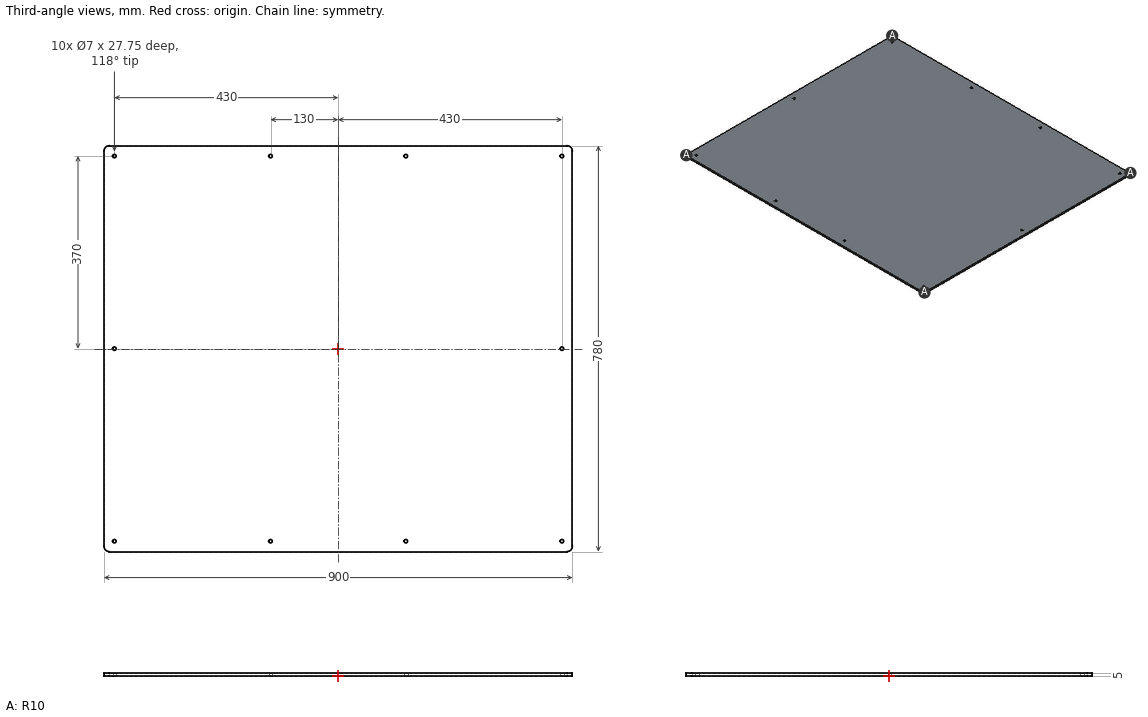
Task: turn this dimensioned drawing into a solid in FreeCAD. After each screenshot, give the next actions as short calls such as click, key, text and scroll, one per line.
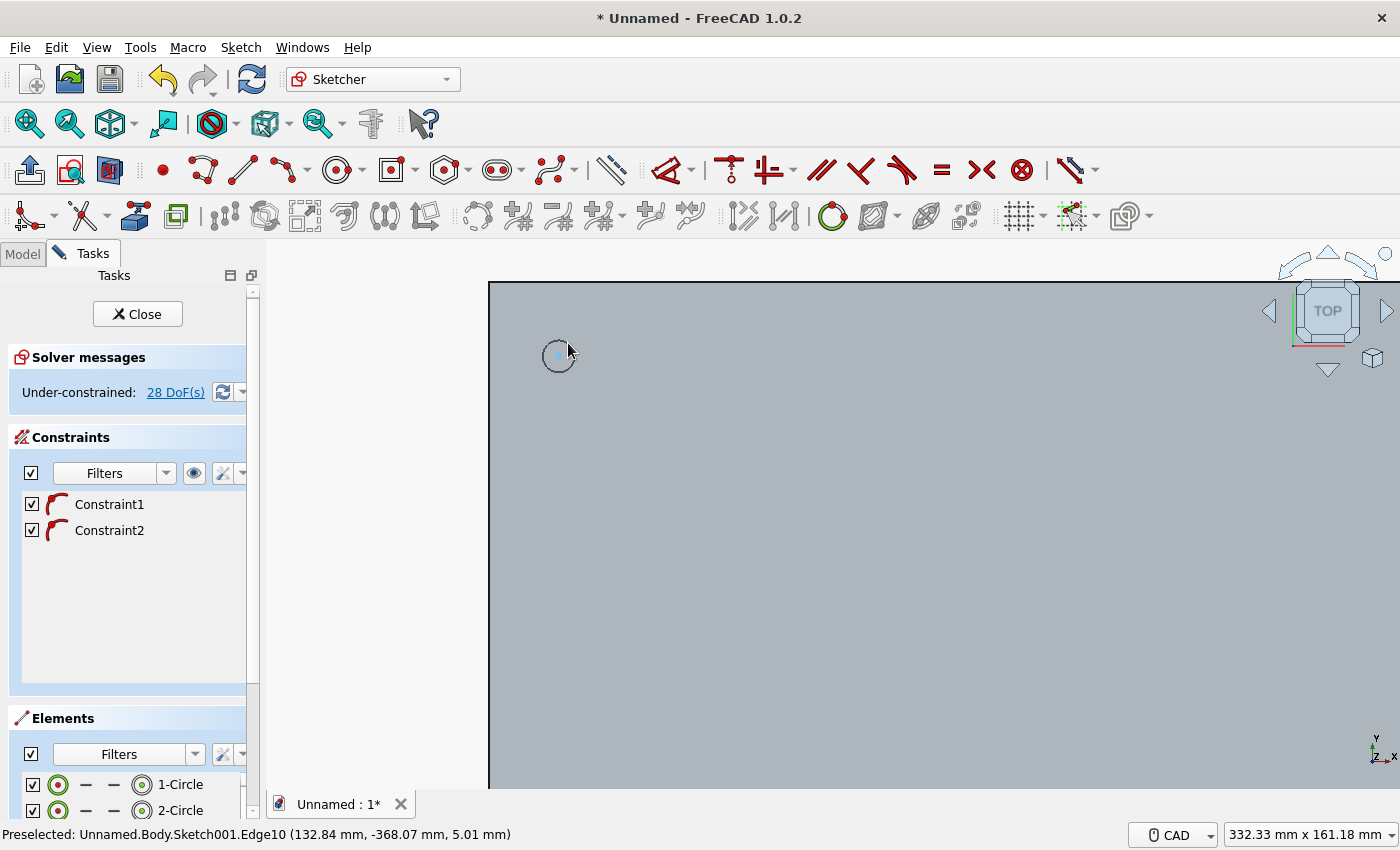
click(570, 345)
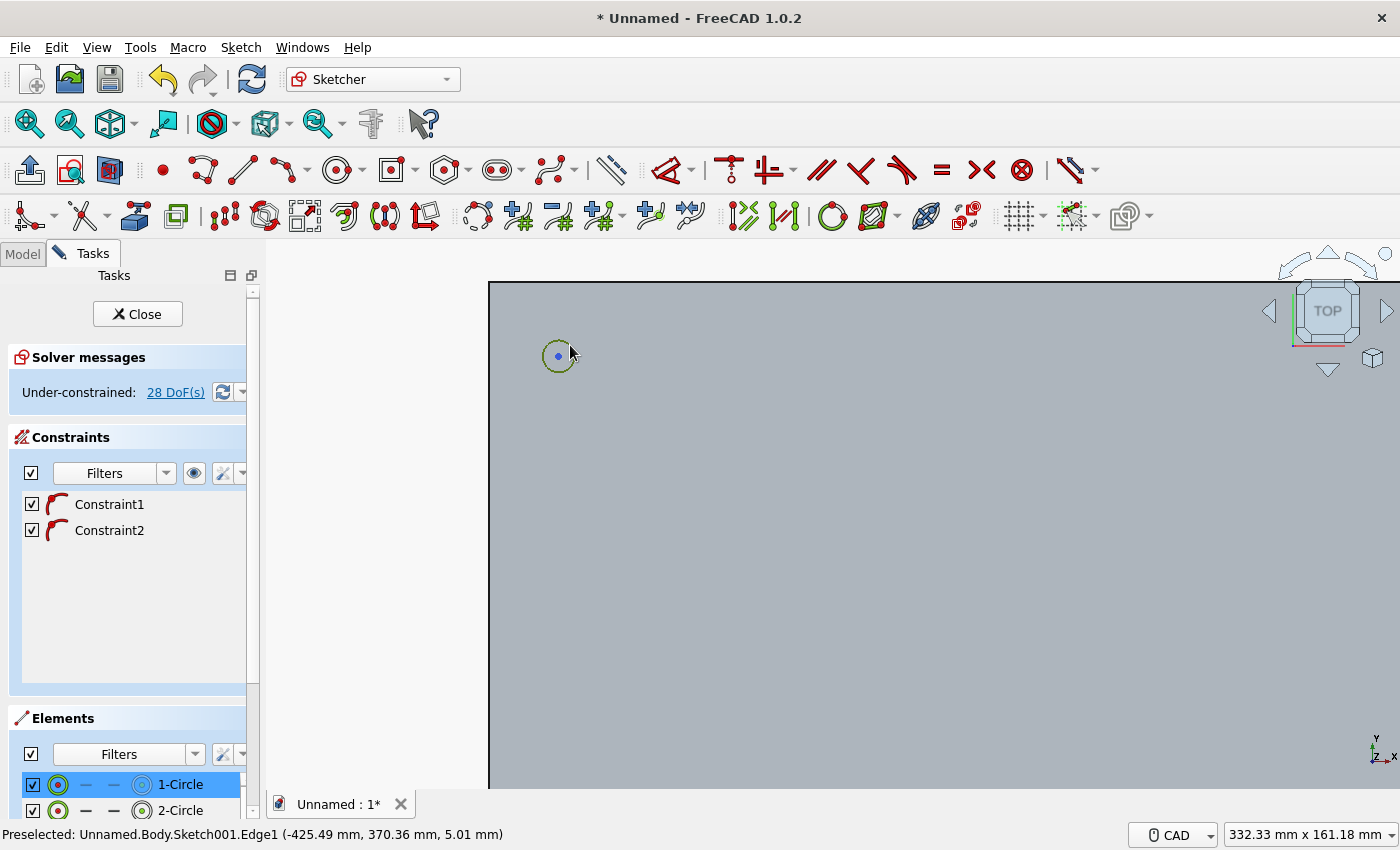
scroll(567, 342, down, 10)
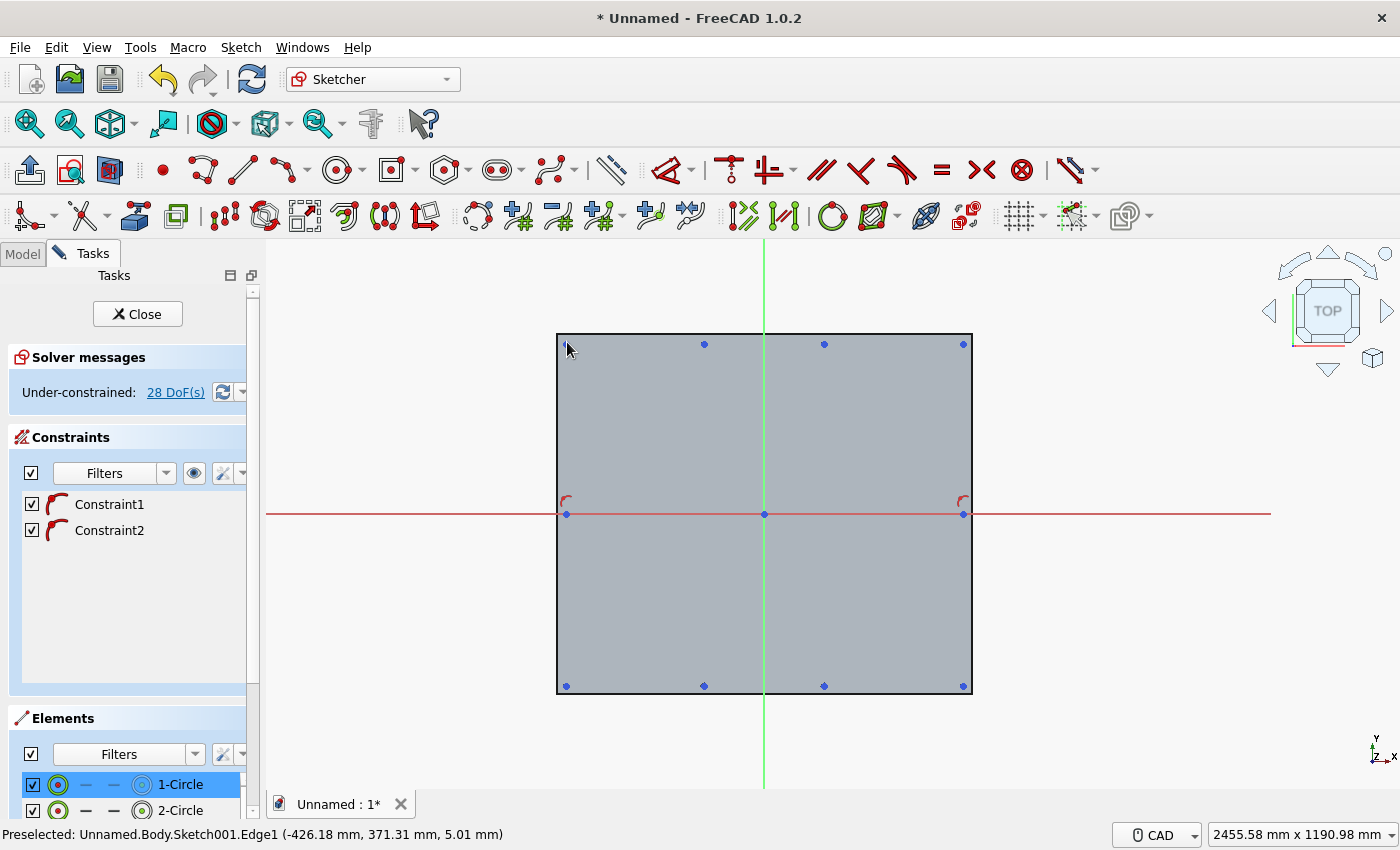
scroll(965, 343, up, 10)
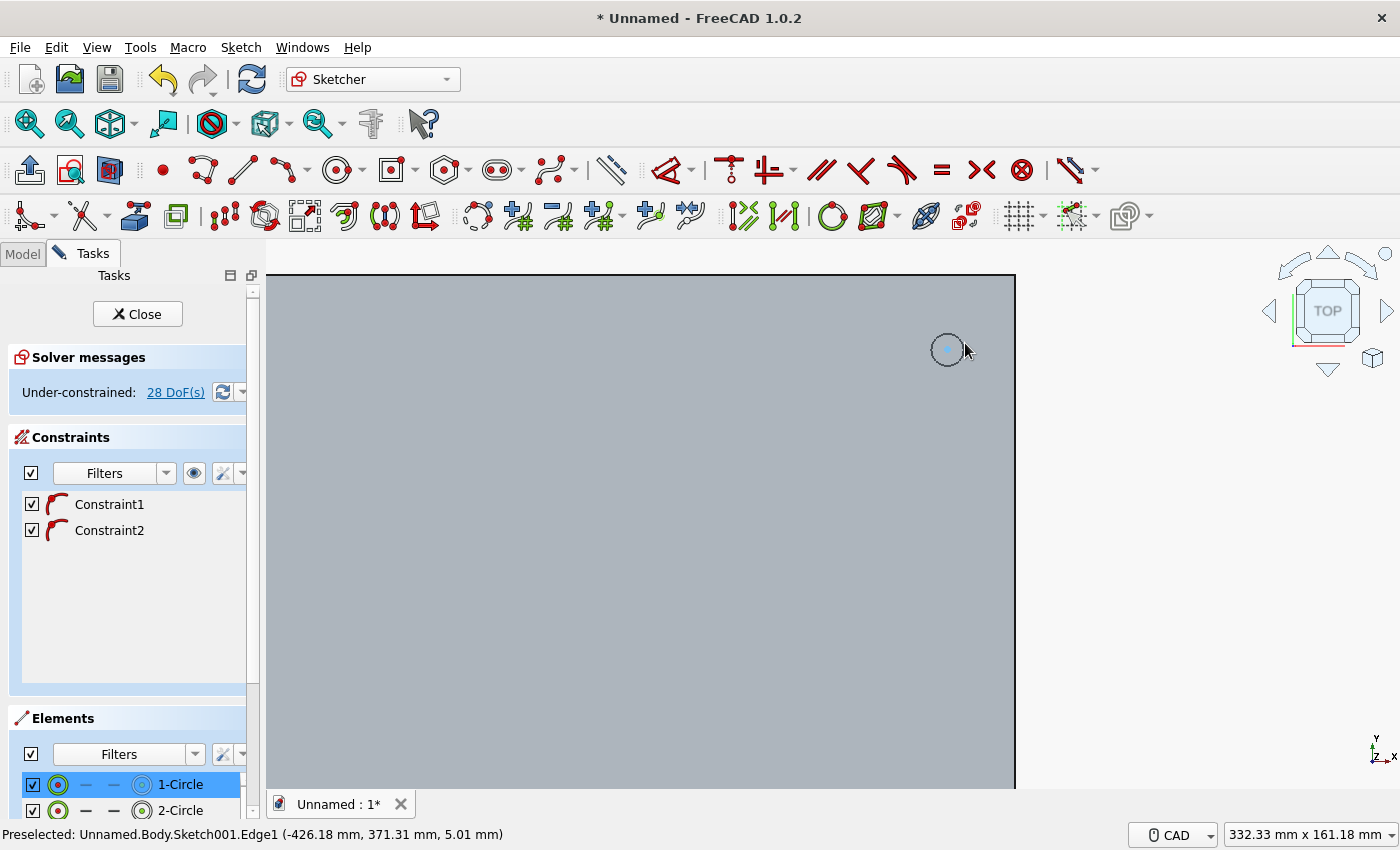
click(959, 339)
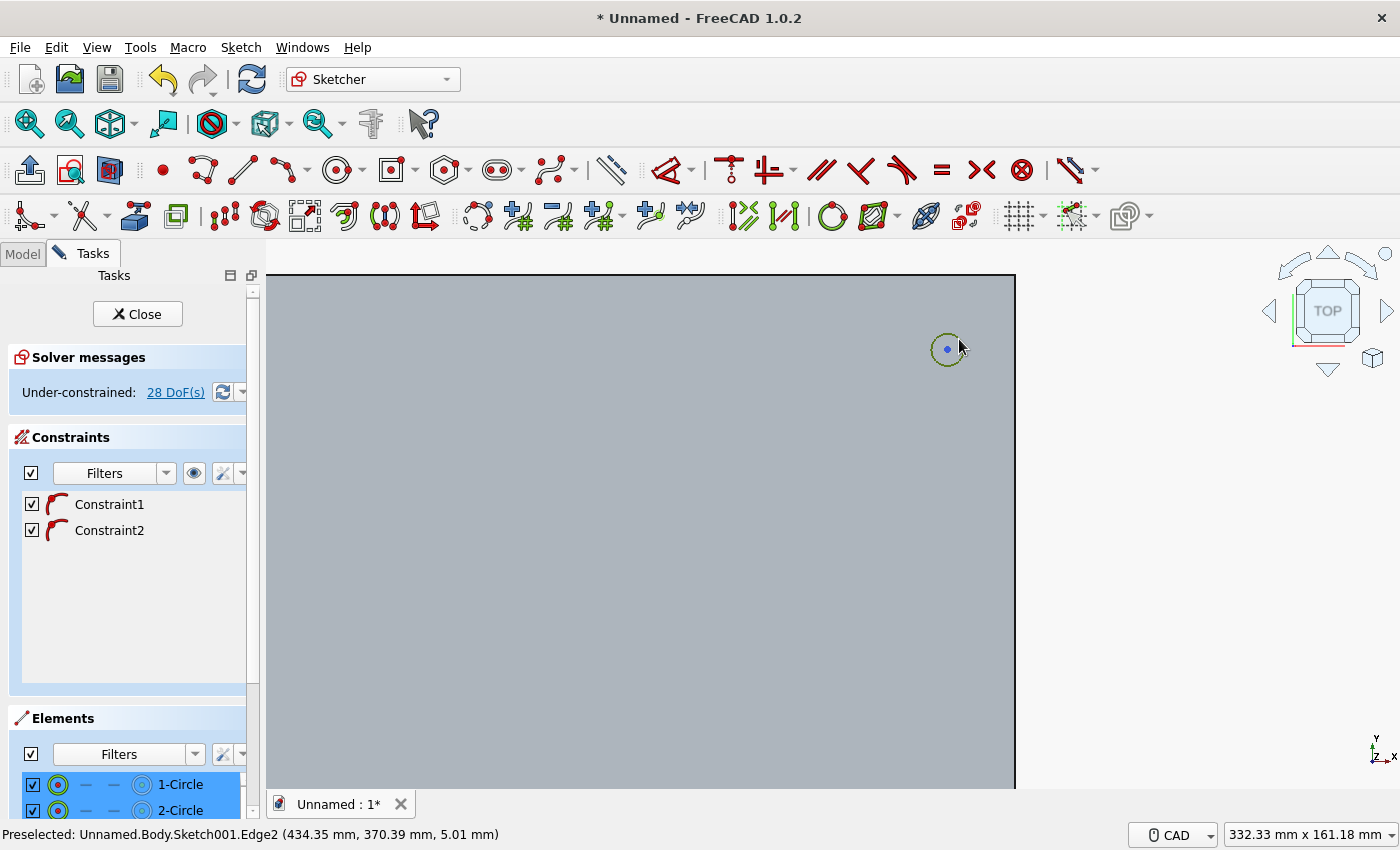
scroll(966, 343, down, 10)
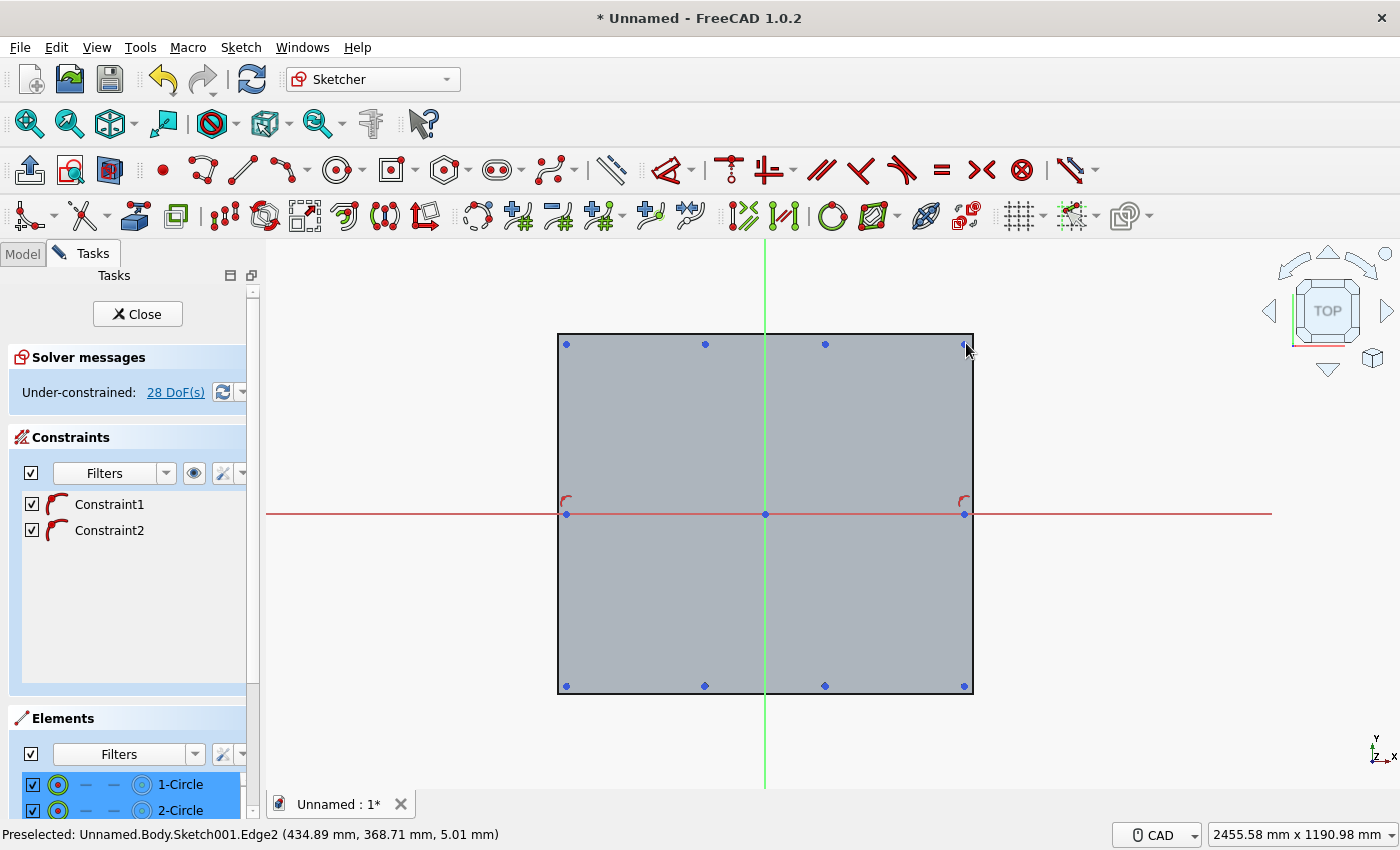
scroll(966, 684, up, 9)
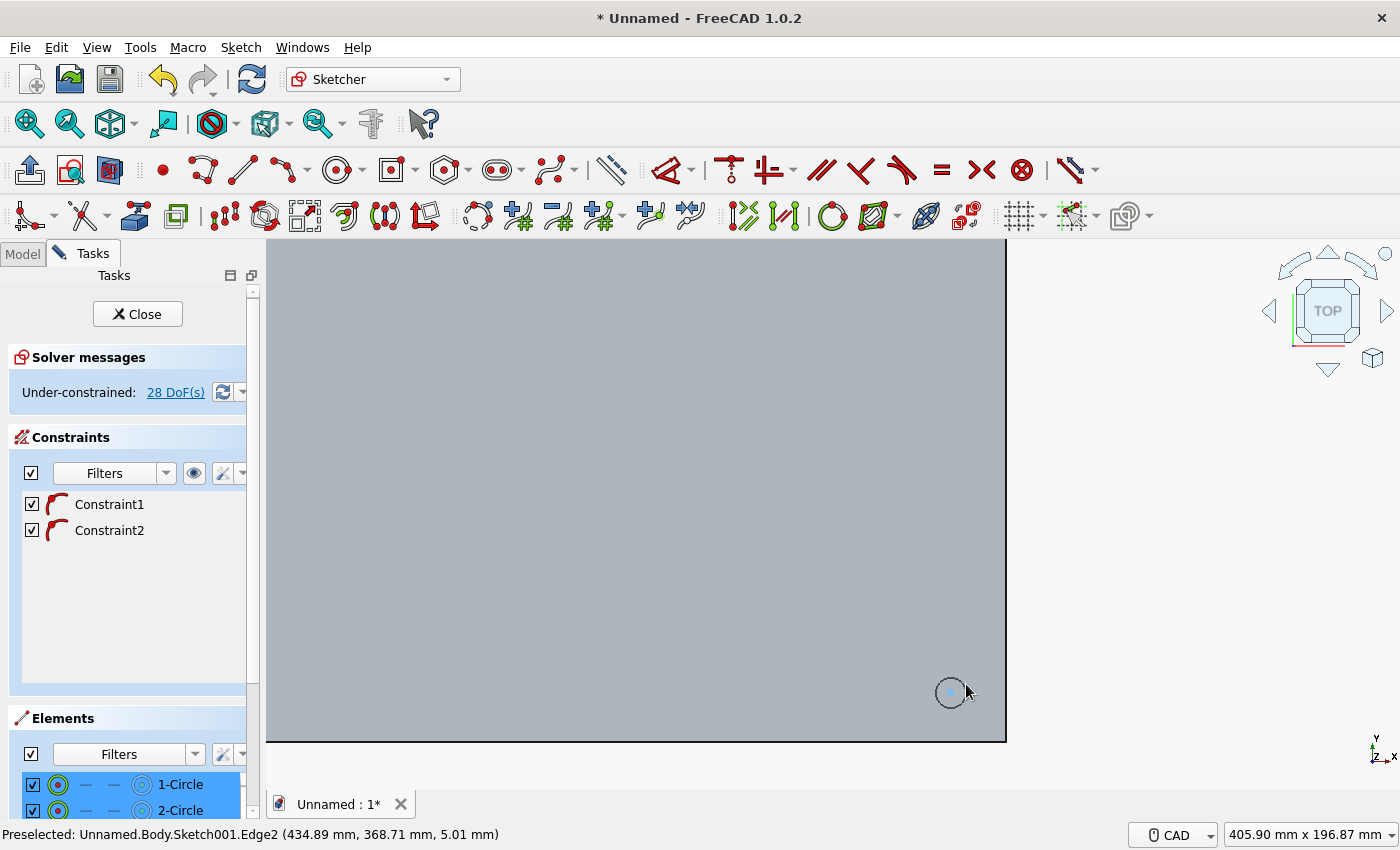
click(962, 682)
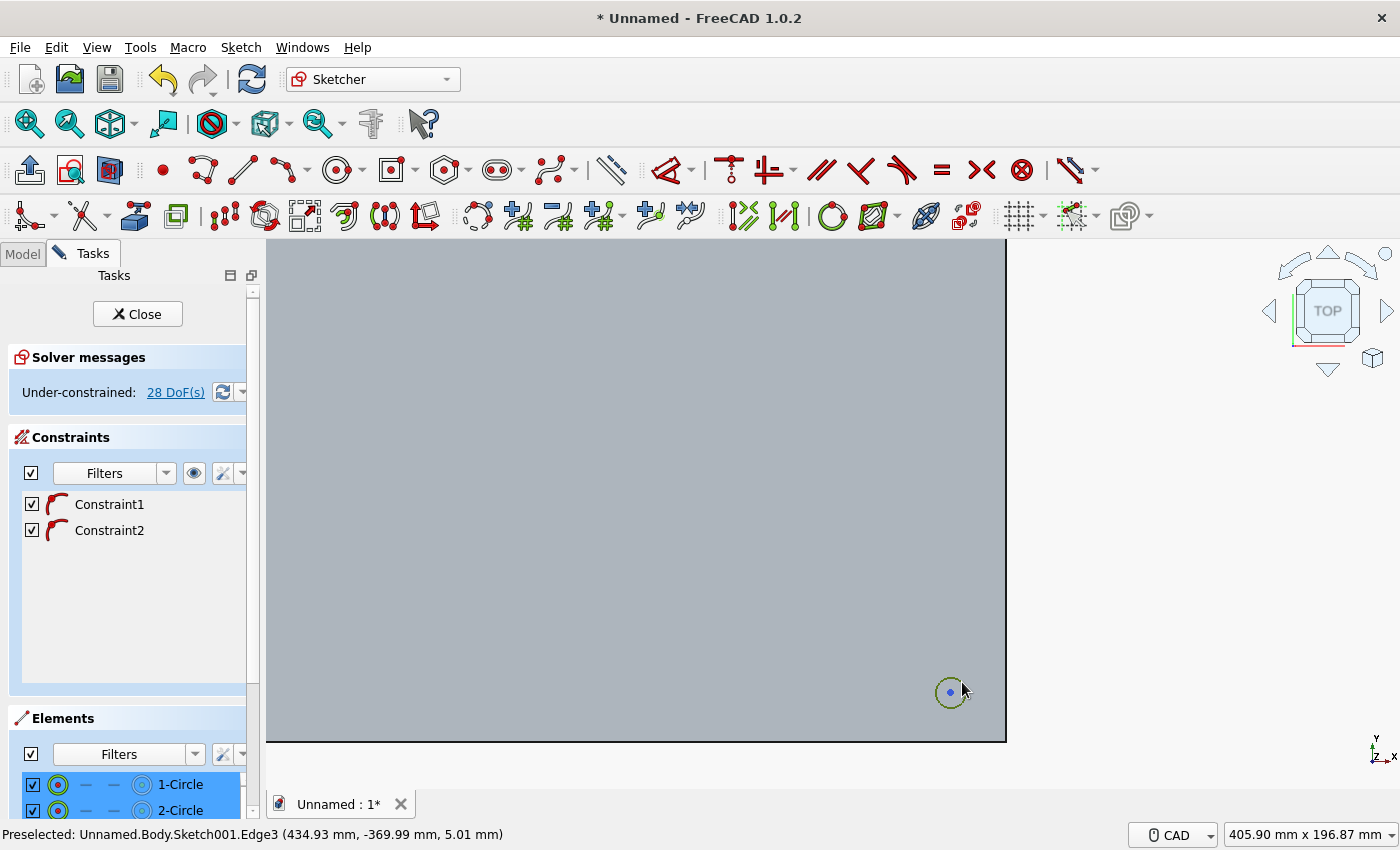
scroll(966, 685, down, 9)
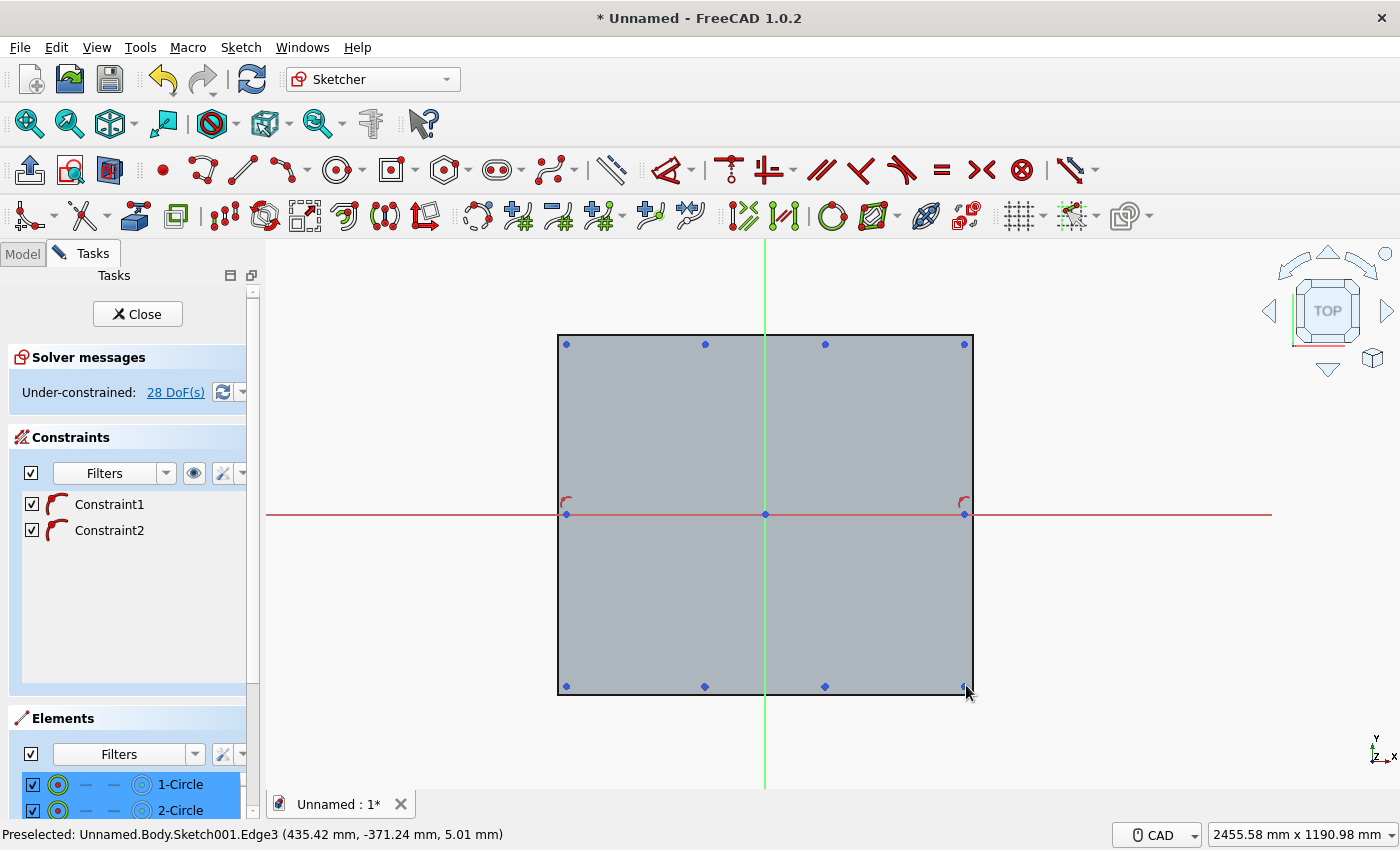
scroll(569, 685, up, 9)